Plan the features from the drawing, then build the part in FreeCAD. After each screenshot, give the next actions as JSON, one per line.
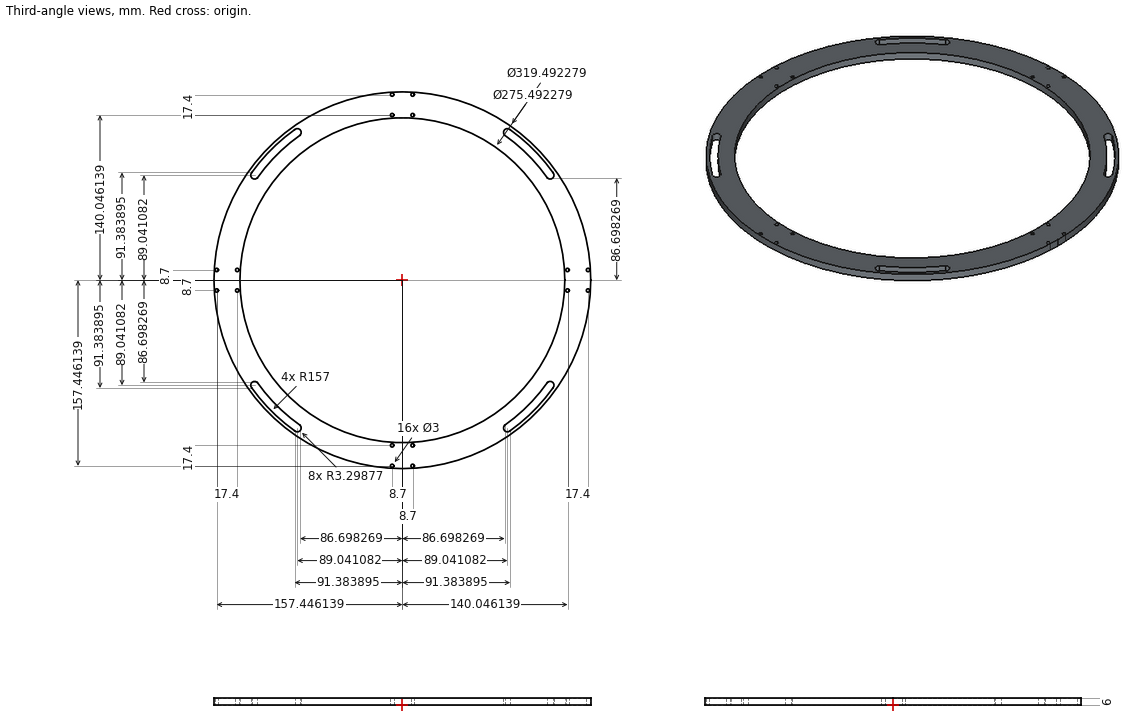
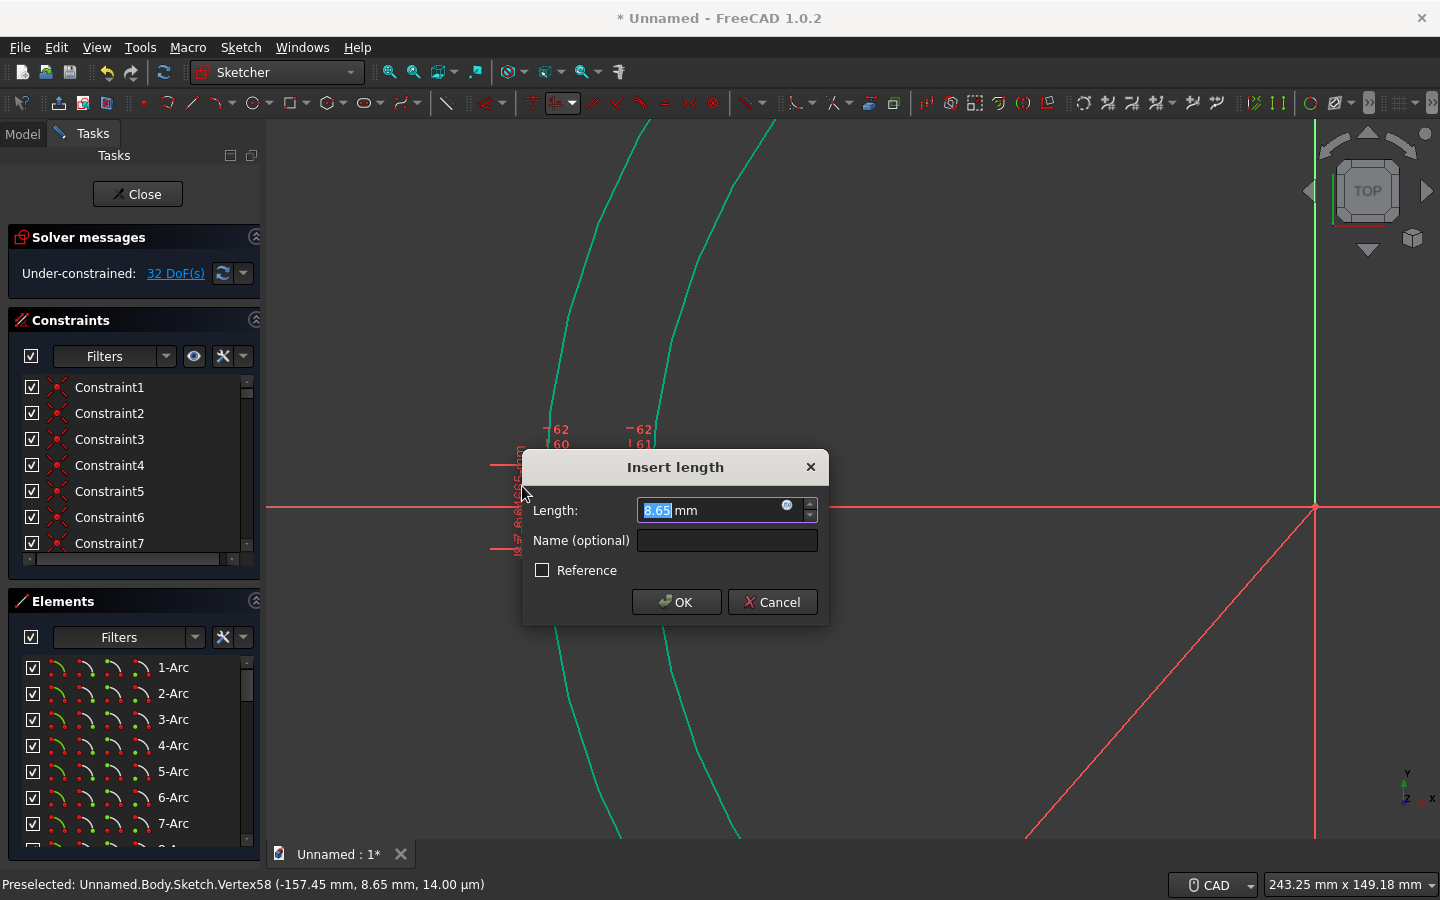
{"action": "type", "text": "8.7"}
{"action": "key", "text": "Return"}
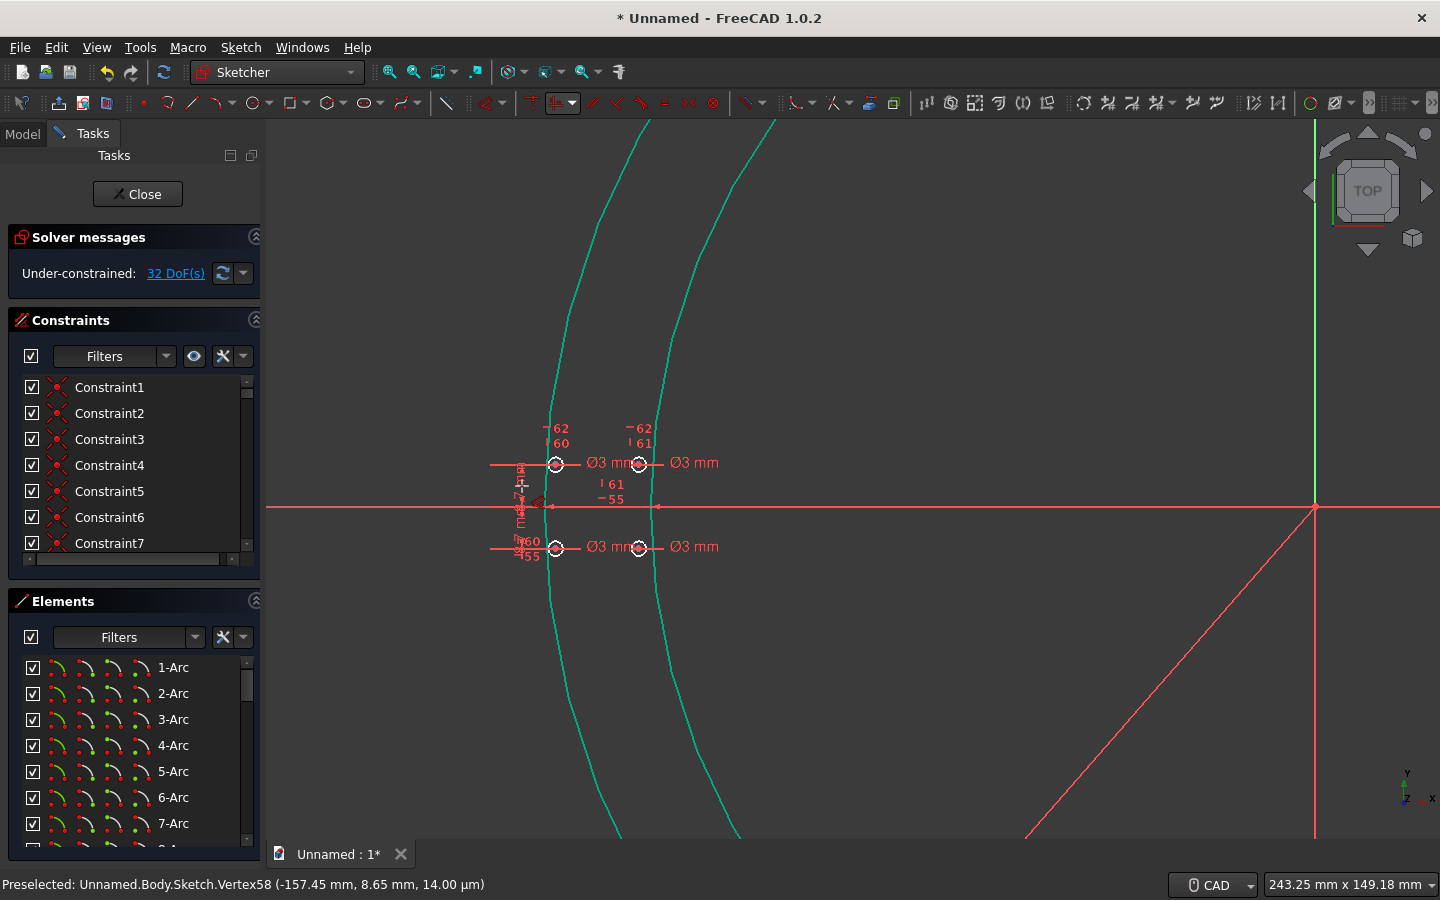
{"action": "scroll", "coordinate": [556, 467], "scroll_direction": "down", "scroll_amount": 6}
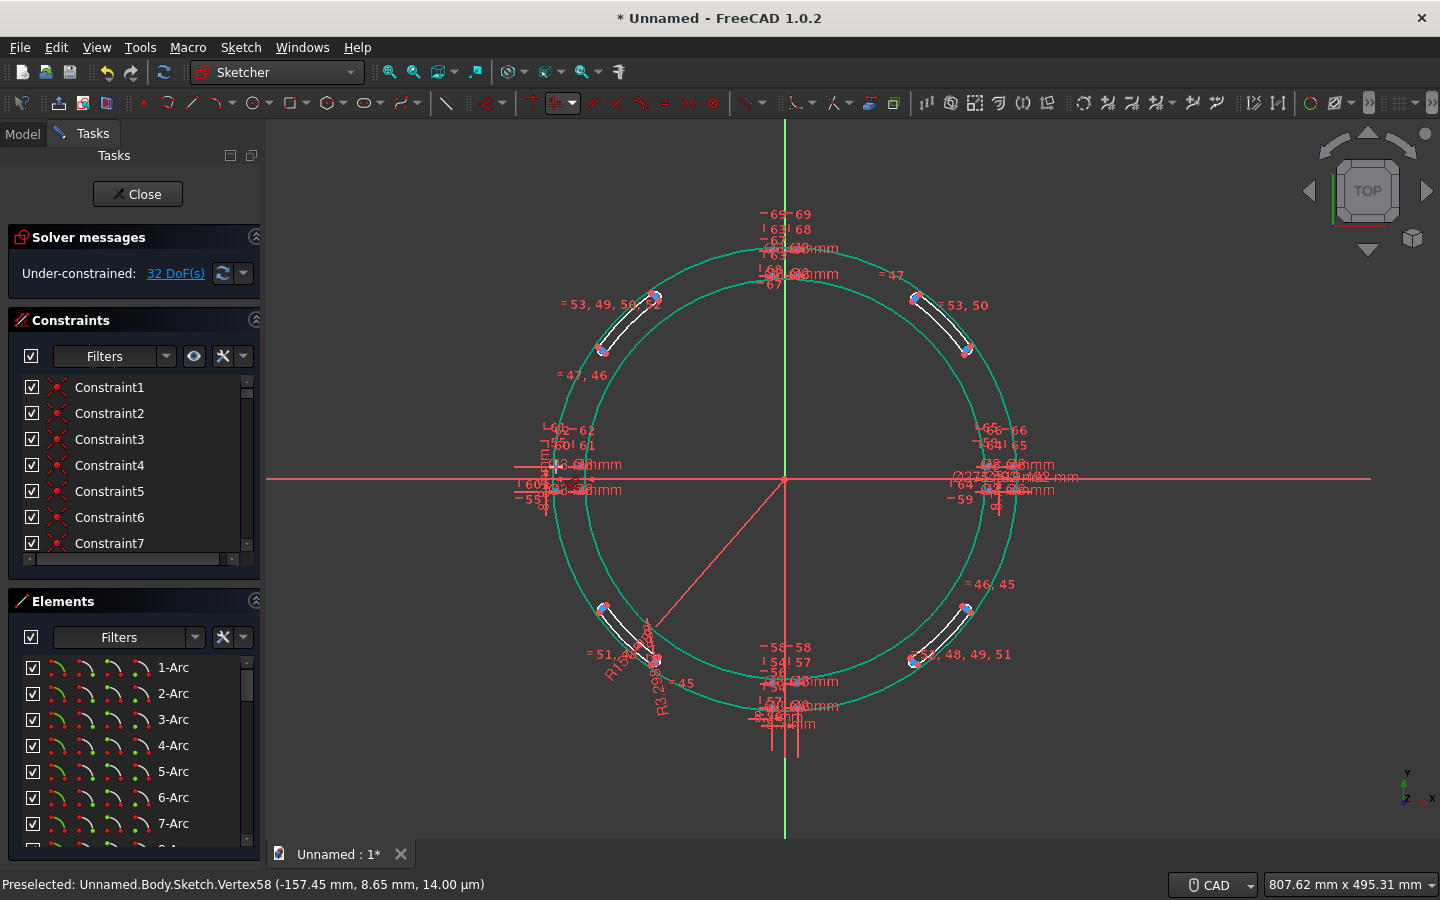
{"action": "scroll", "coordinate": [772, 276], "scroll_direction": "up", "scroll_amount": 6}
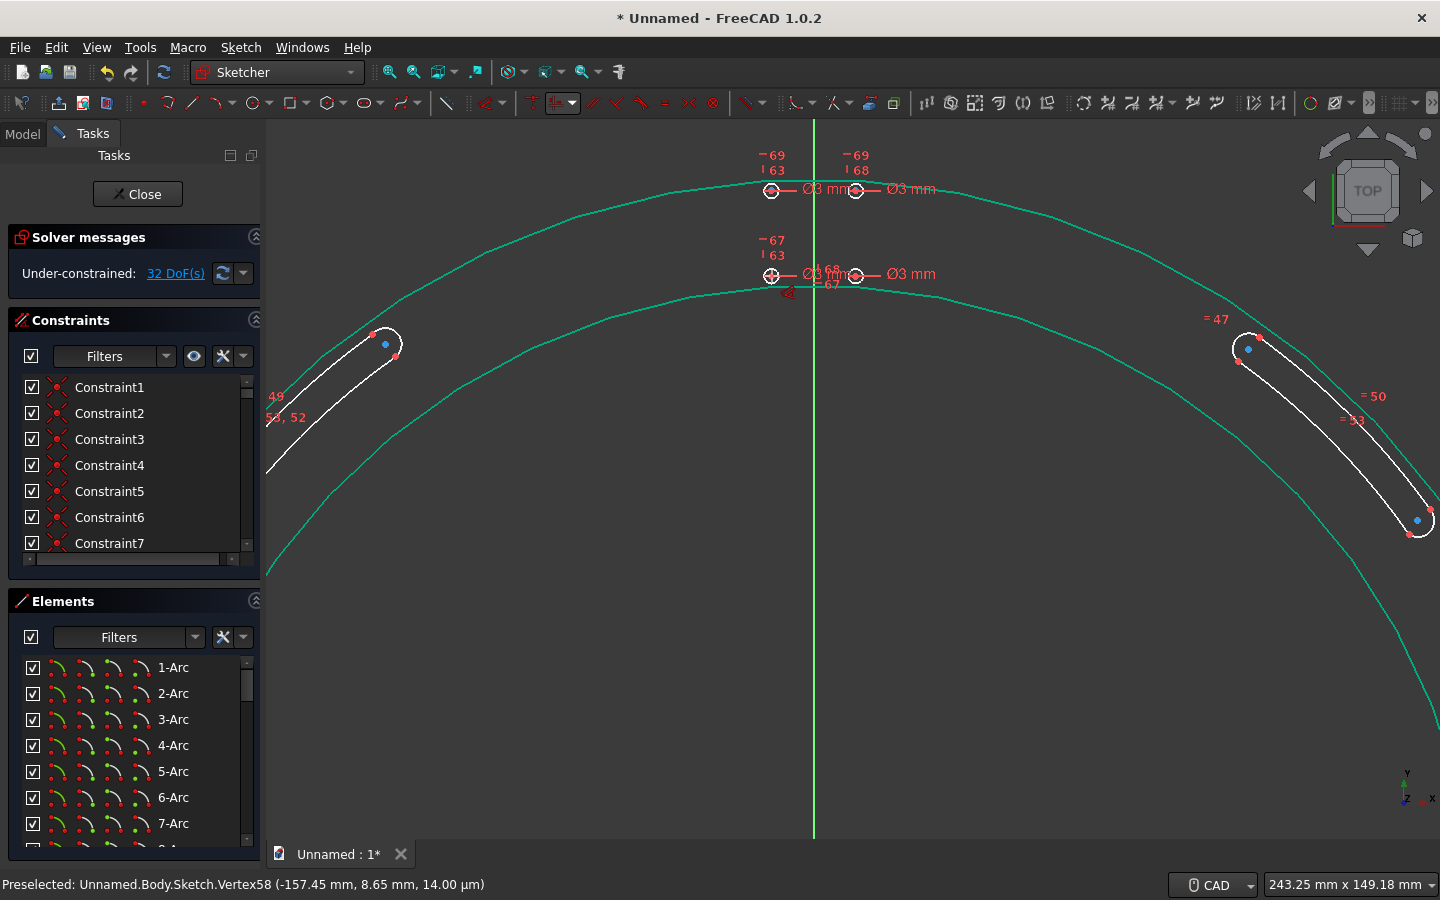
{"action": "left_click", "coordinate": [771, 276]}
{"action": "left_click", "coordinate": [793, 242]}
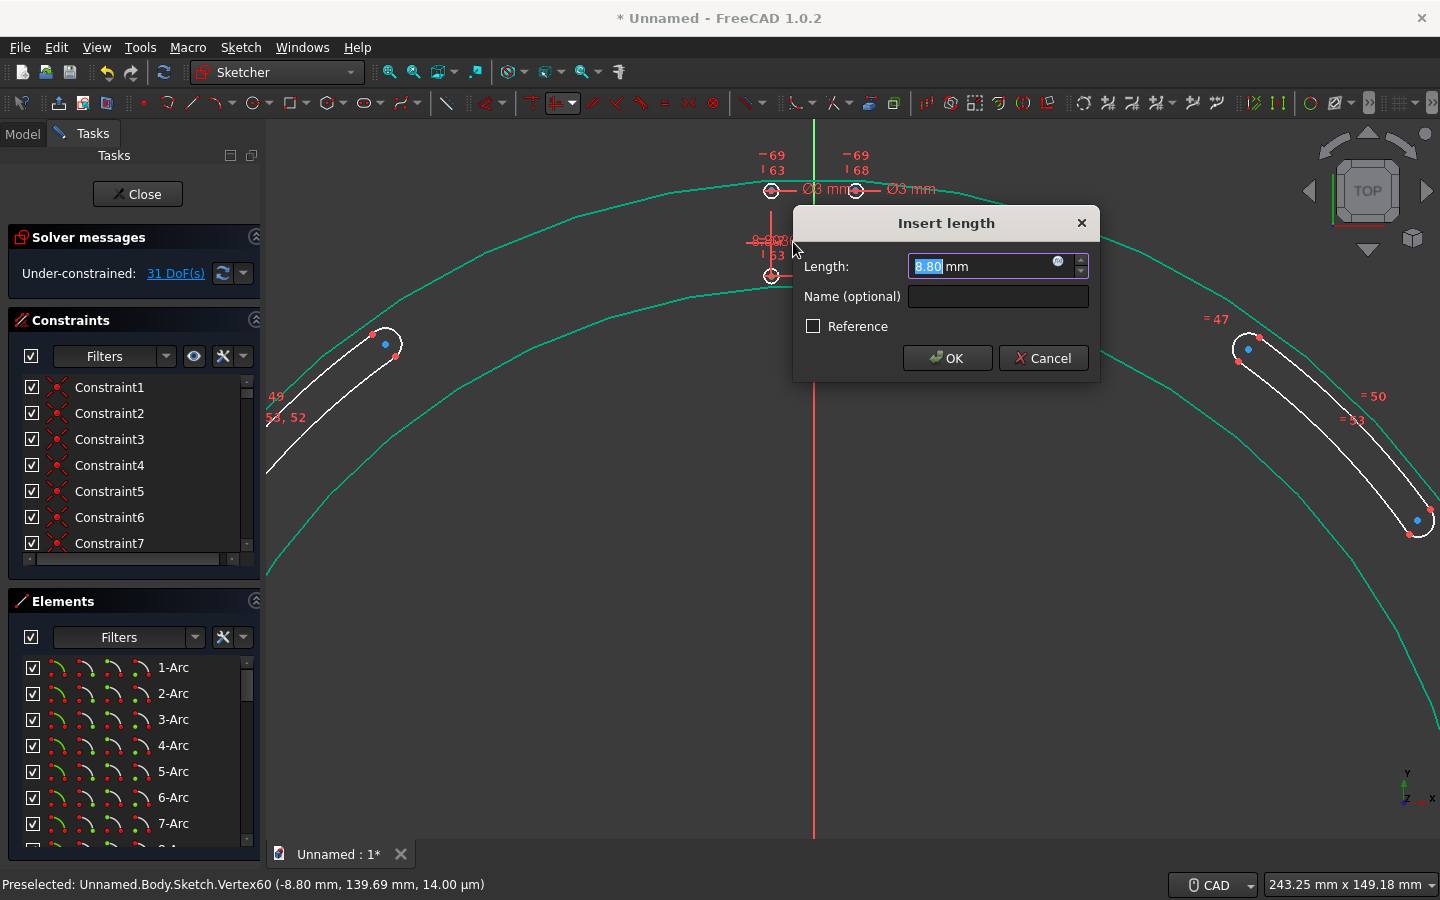
{"action": "type", "text": "8.7"}
{"action": "key", "text": "Return"}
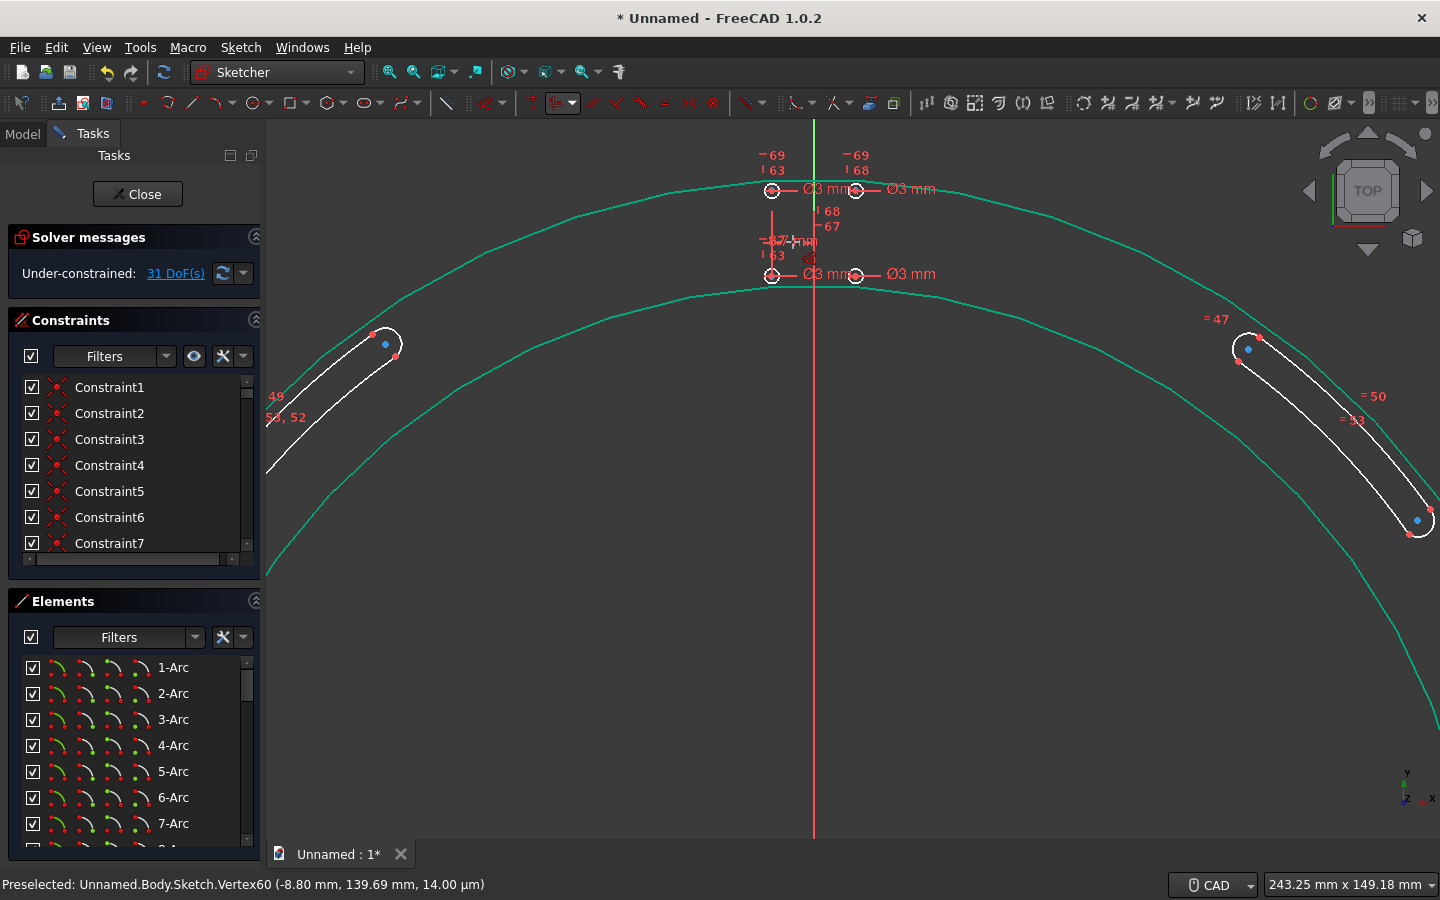
{"action": "scroll", "coordinate": [772, 276], "scroll_direction": "down", "scroll_amount": 6}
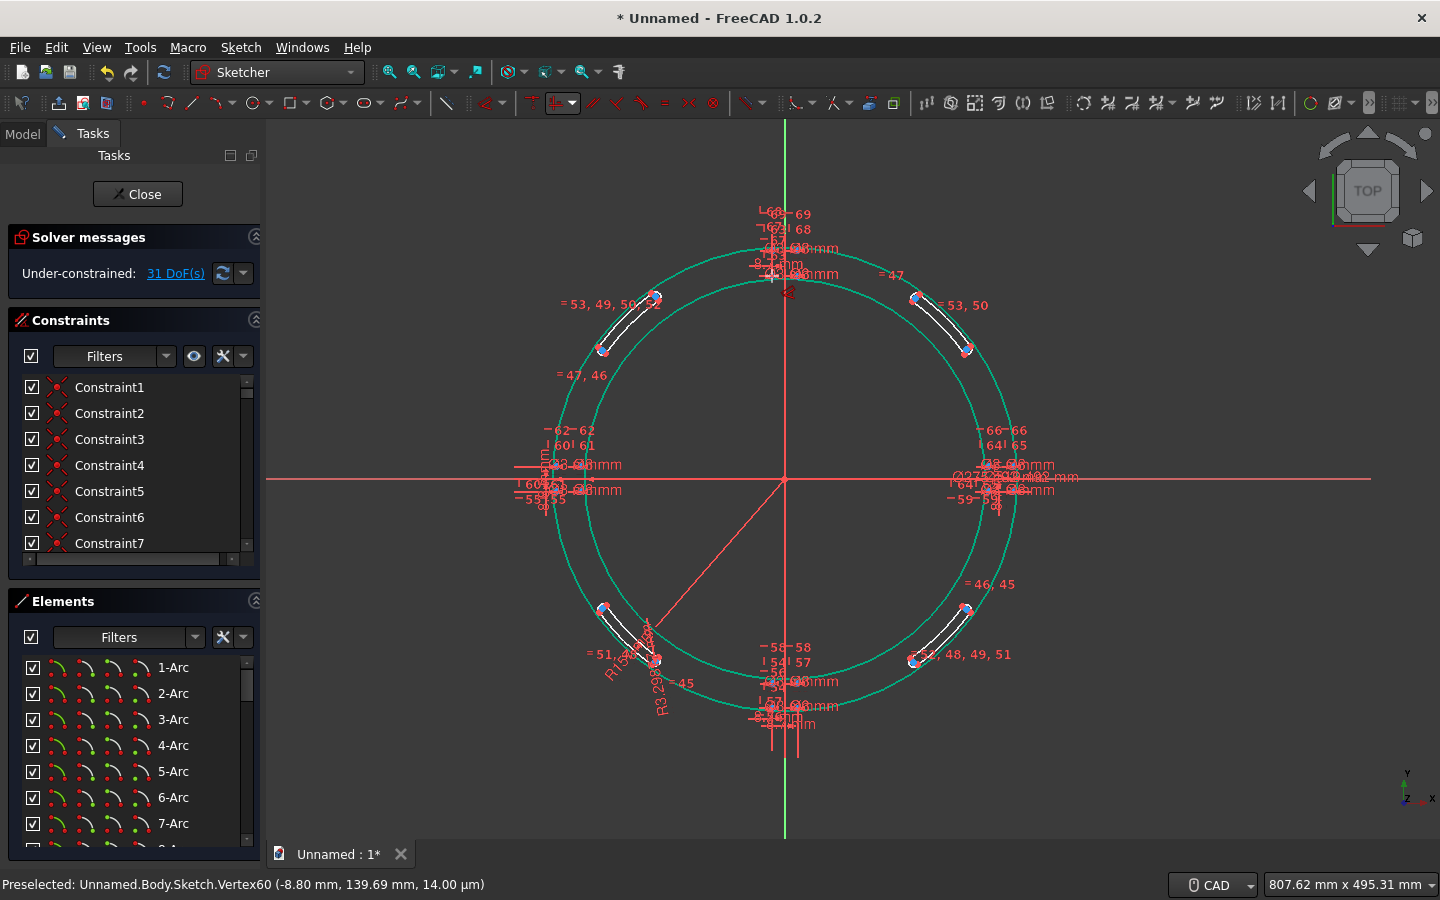
{"action": "scroll", "coordinate": [988, 467], "scroll_direction": "up", "scroll_amount": 6}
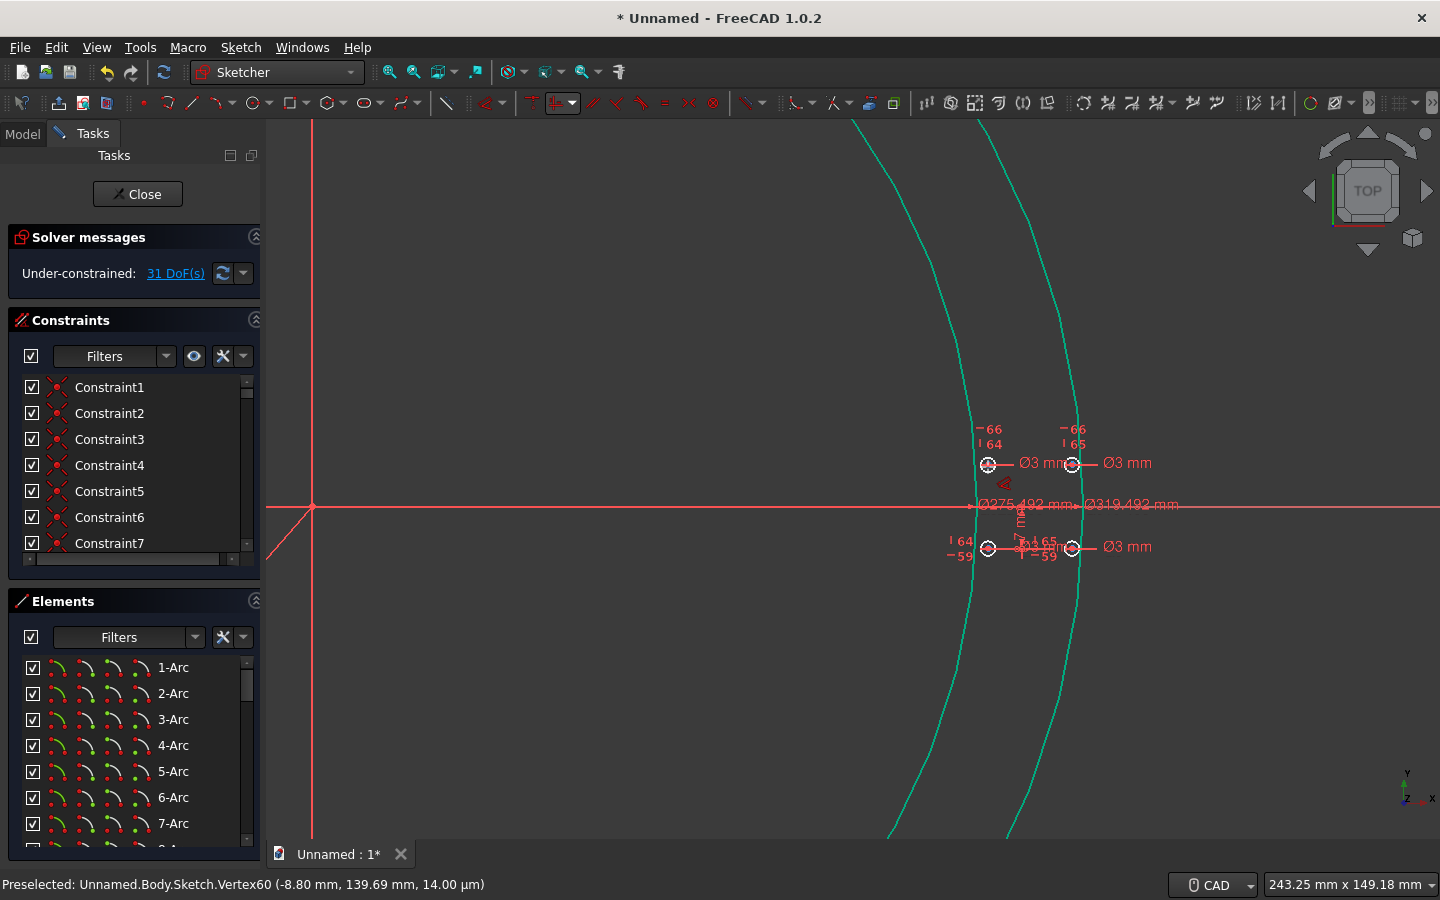
{"action": "left_click", "coordinate": [988, 465]}
{"action": "left_click", "coordinate": [1022, 486]}